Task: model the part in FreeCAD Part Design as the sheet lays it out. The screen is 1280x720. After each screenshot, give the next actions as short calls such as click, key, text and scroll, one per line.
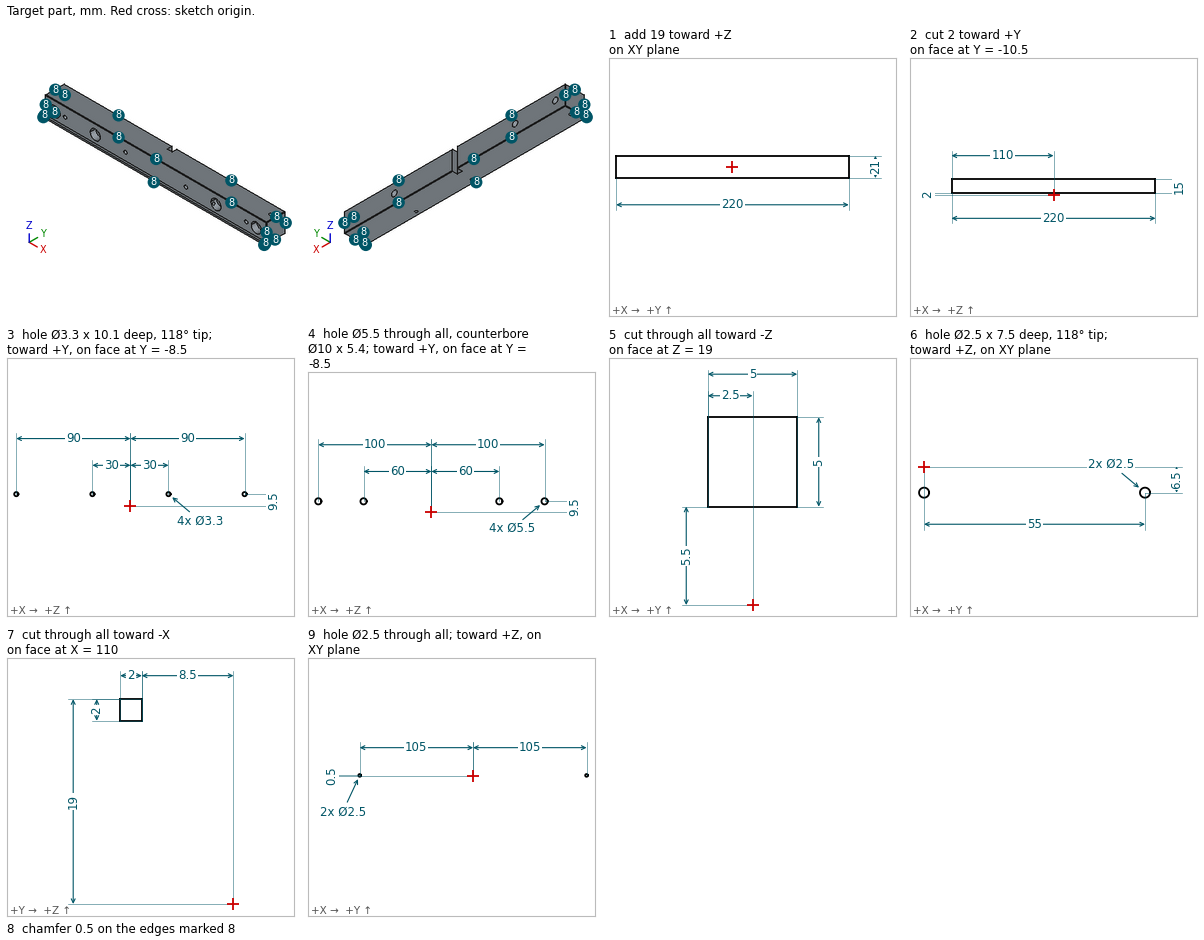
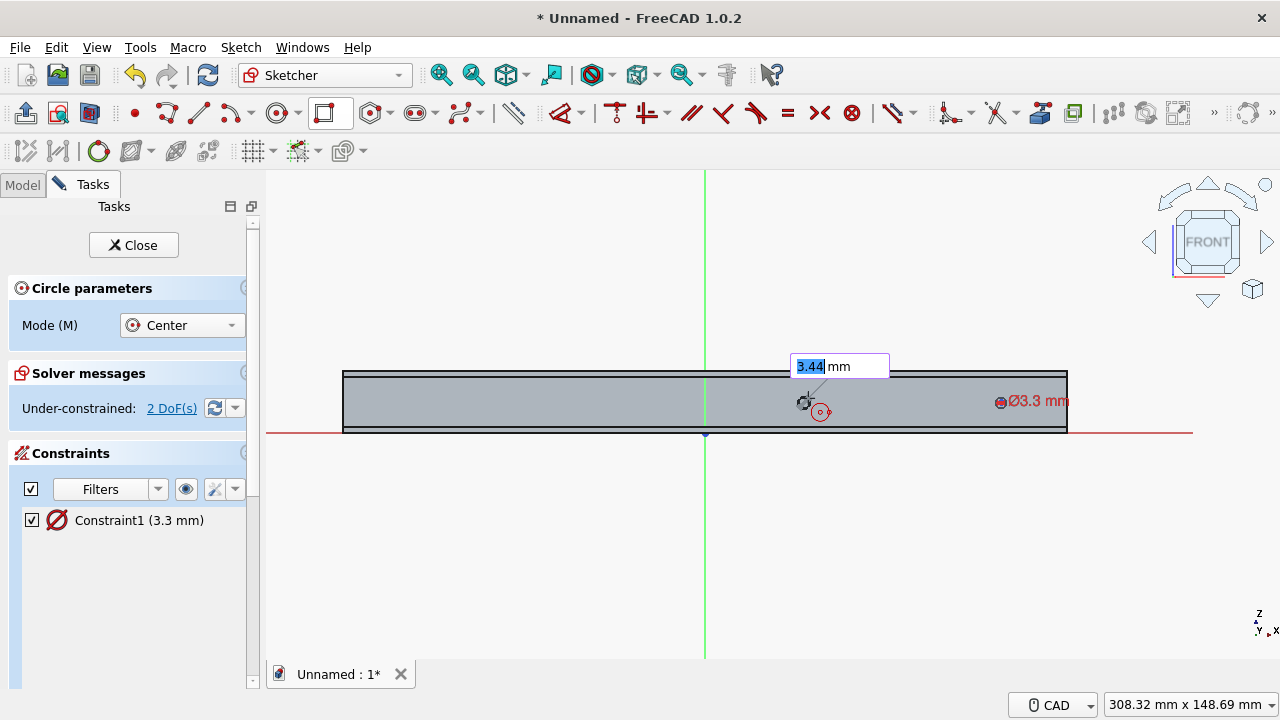
text(3.3)
key(Return)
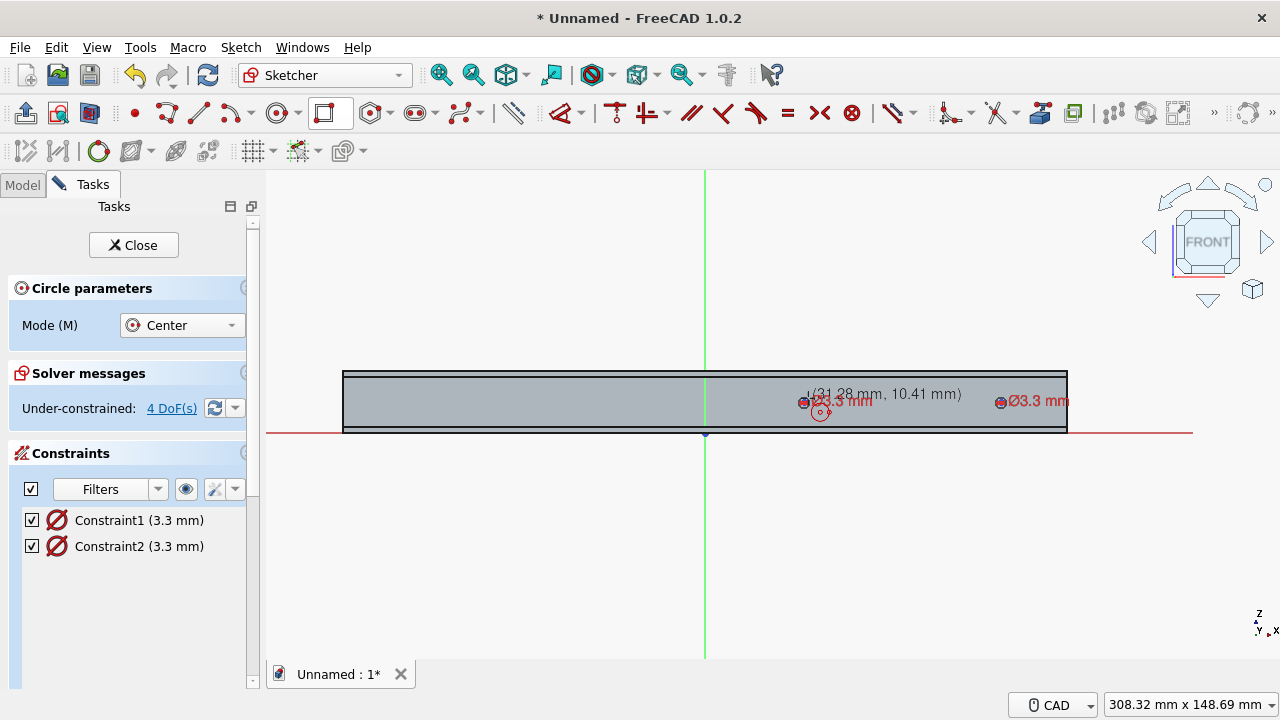
scroll(606, 402, up, 8)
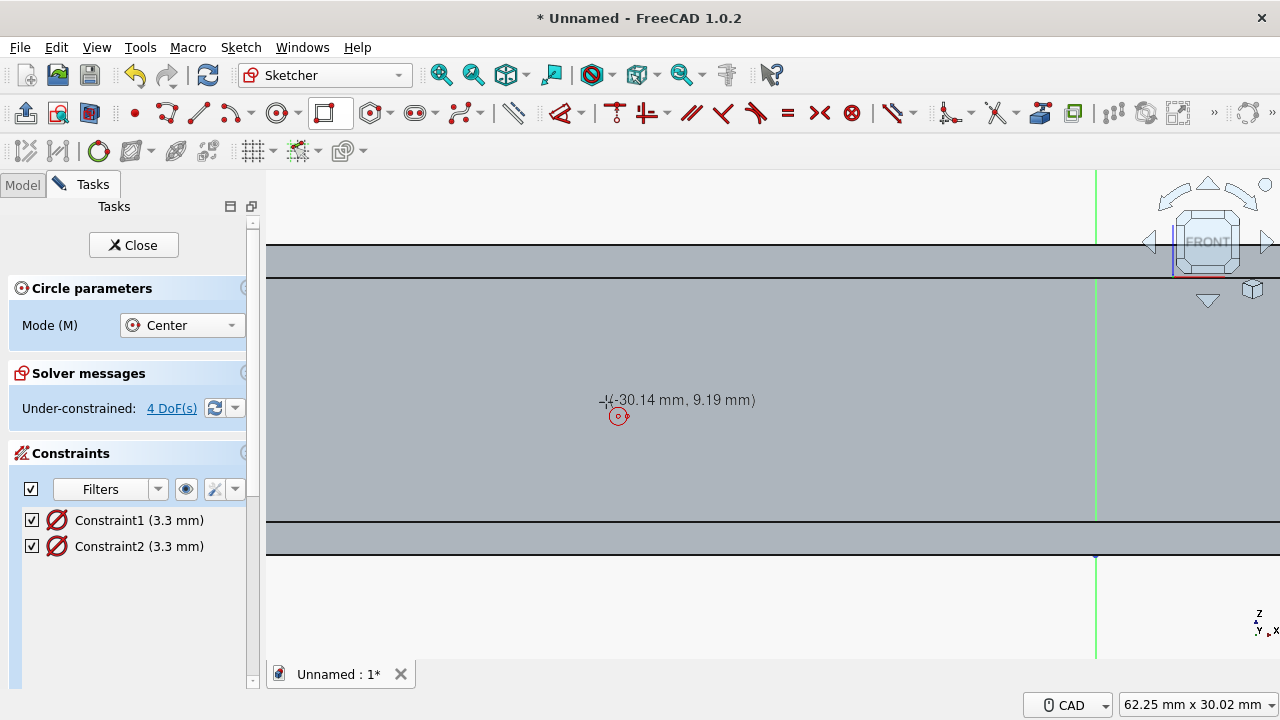
scroll(606, 402, down, 8)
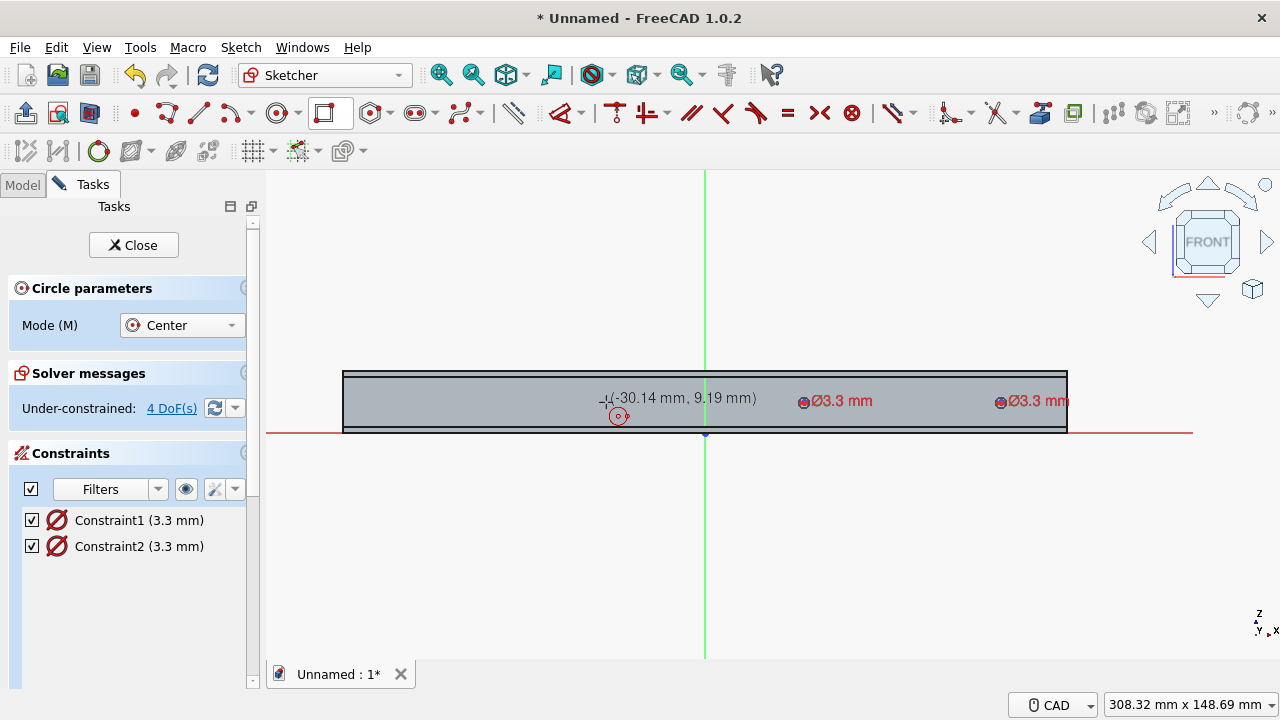
click(606, 402)
move(610, 398)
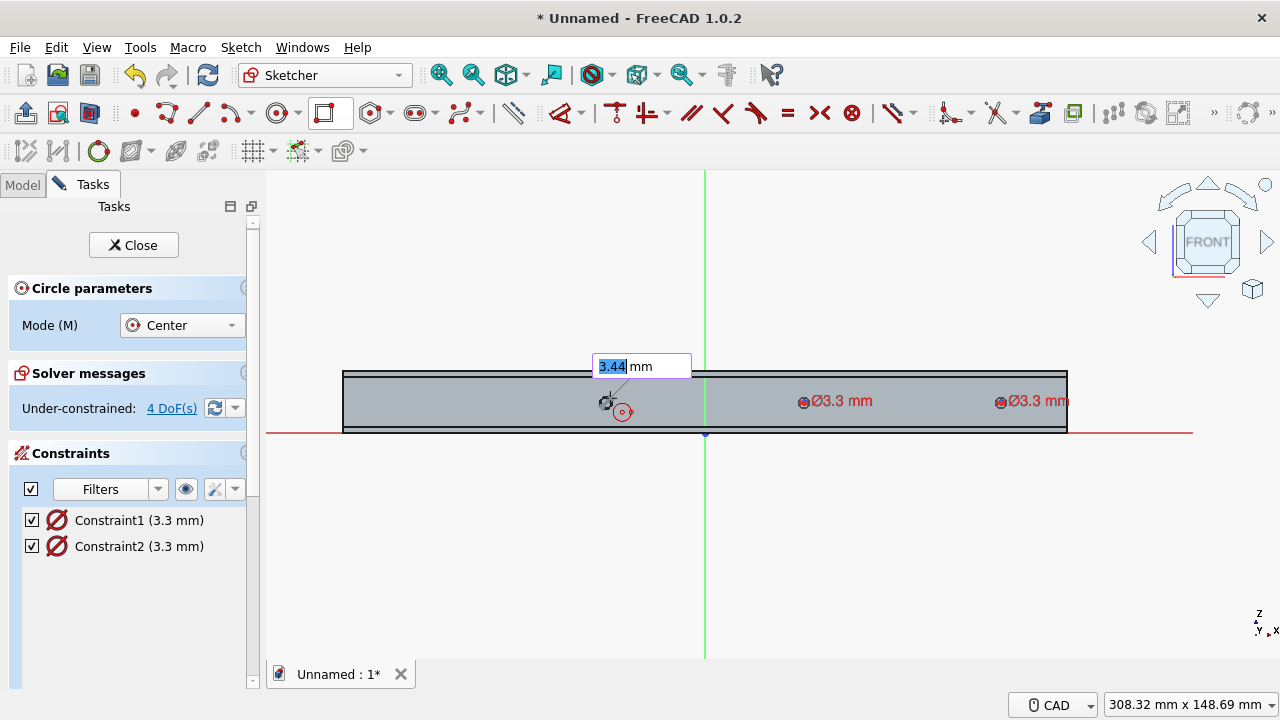
text(3.3)
key(Return)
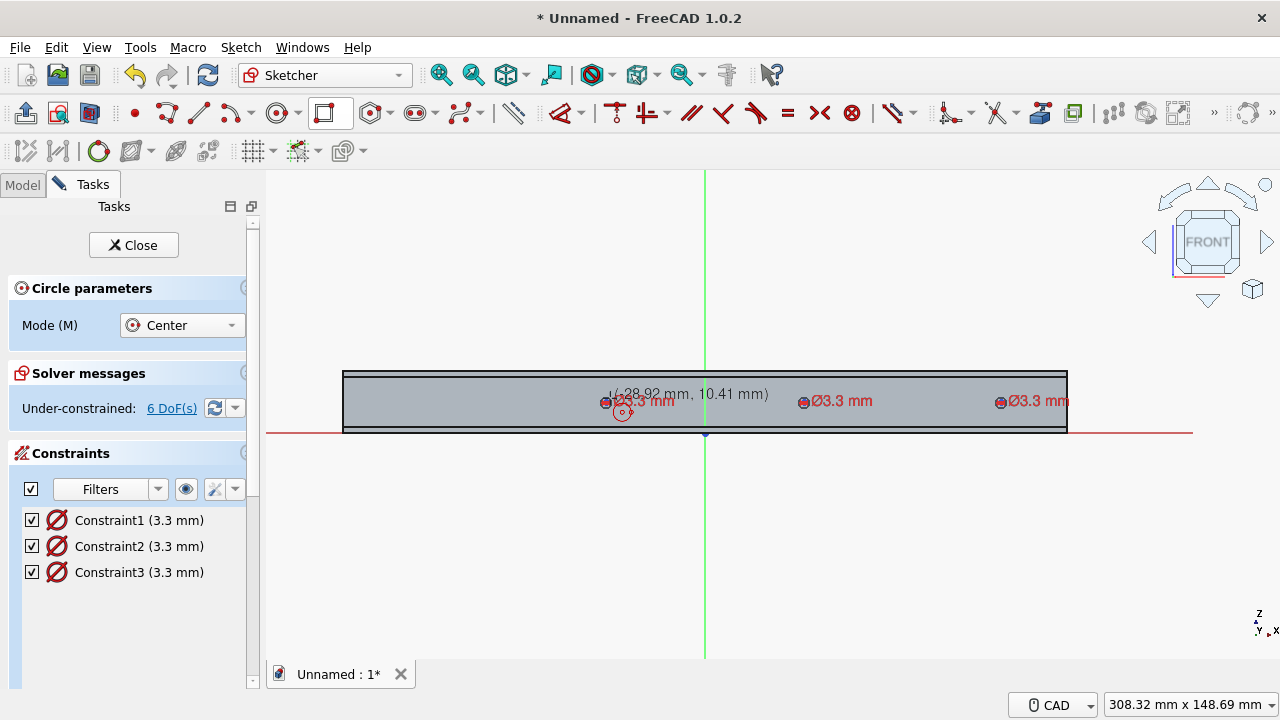
scroll(409, 402, up, 8)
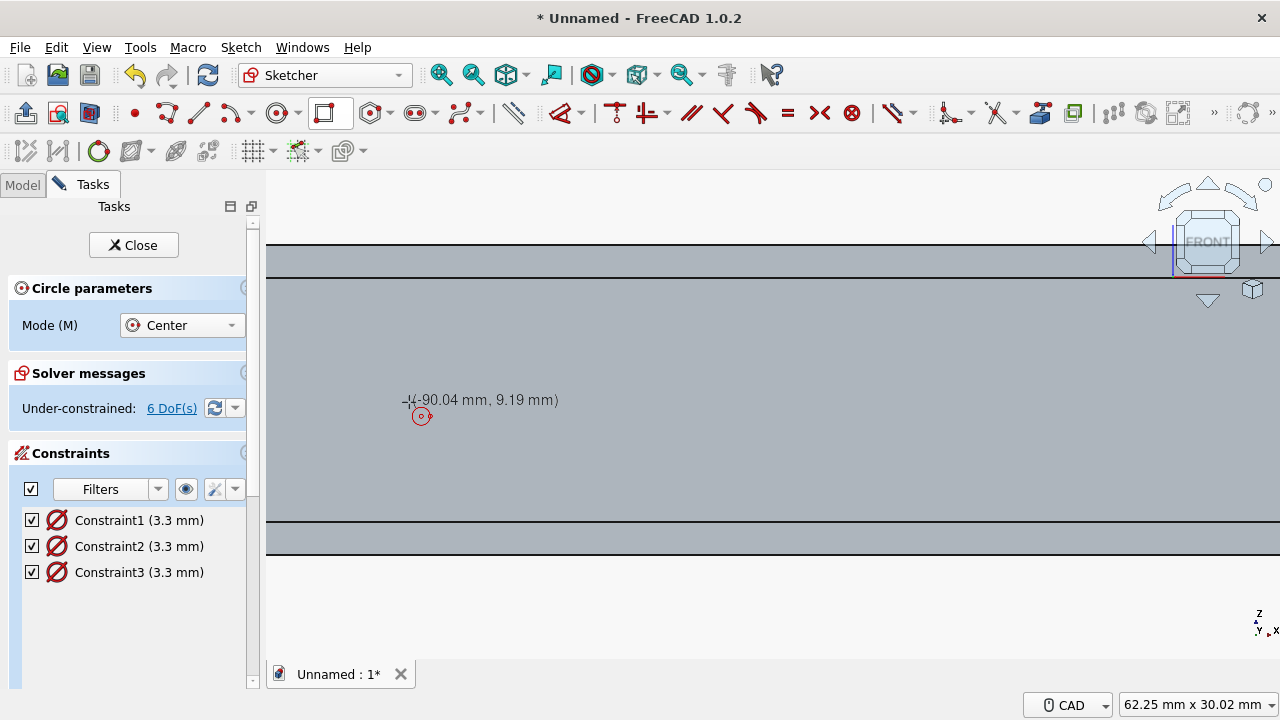
scroll(408, 402, down, 8)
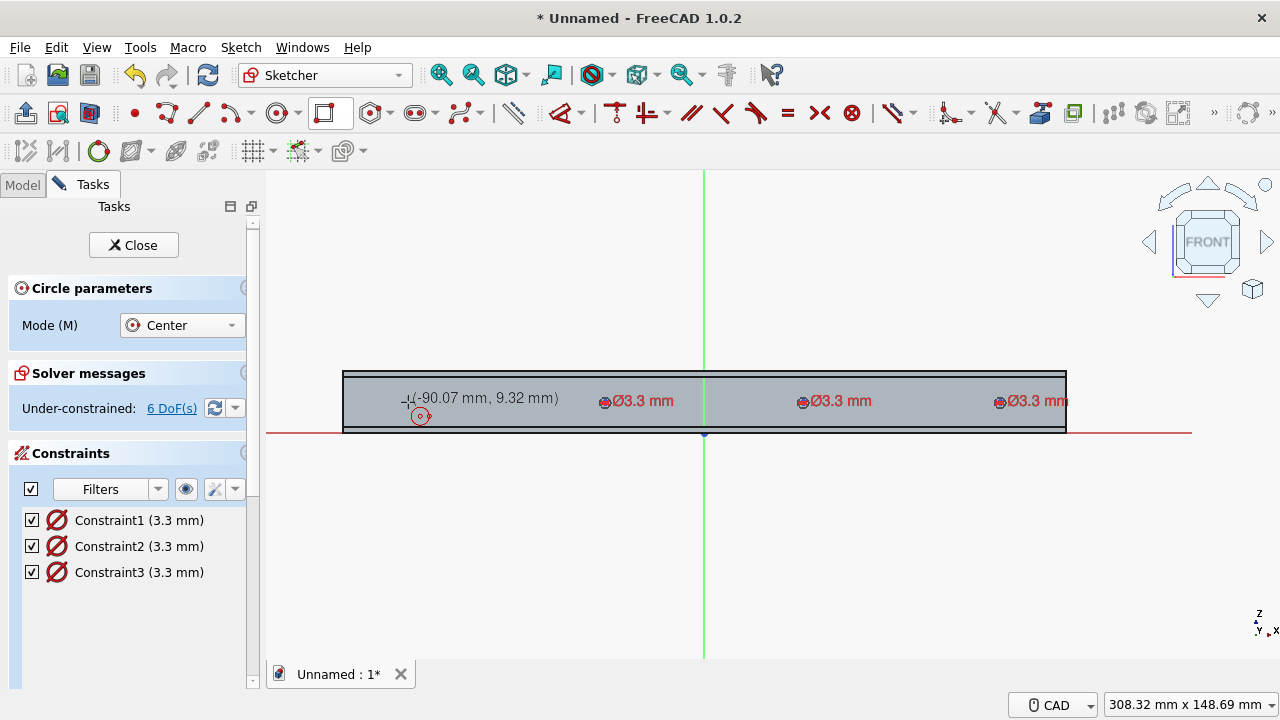
click(408, 402)
move(412, 398)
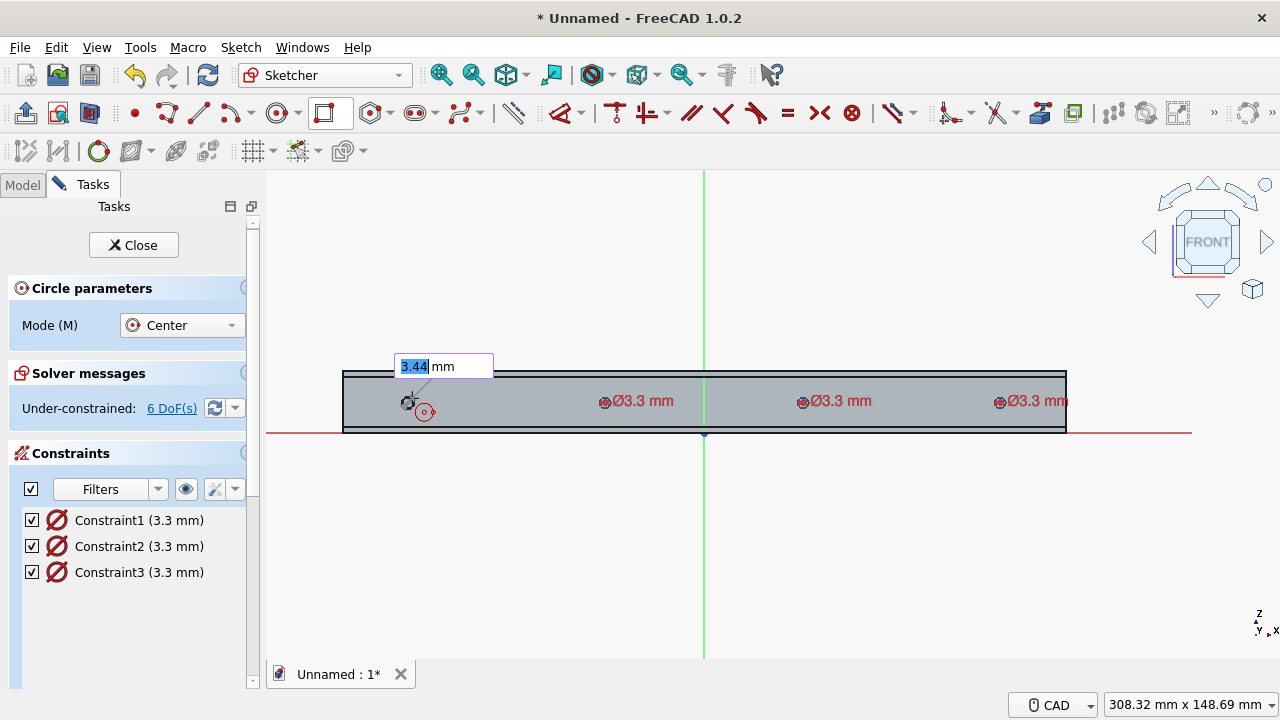
text(3.3)
key(Return)
key(Escape)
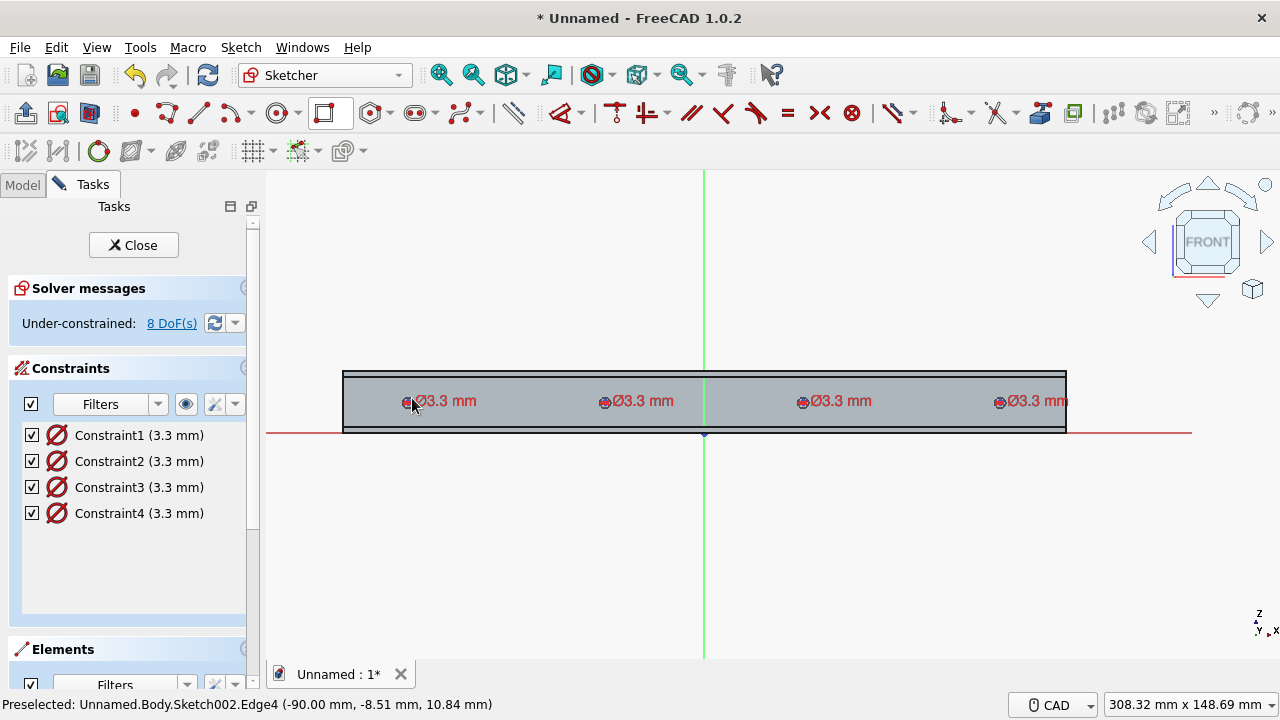
click(1000, 403)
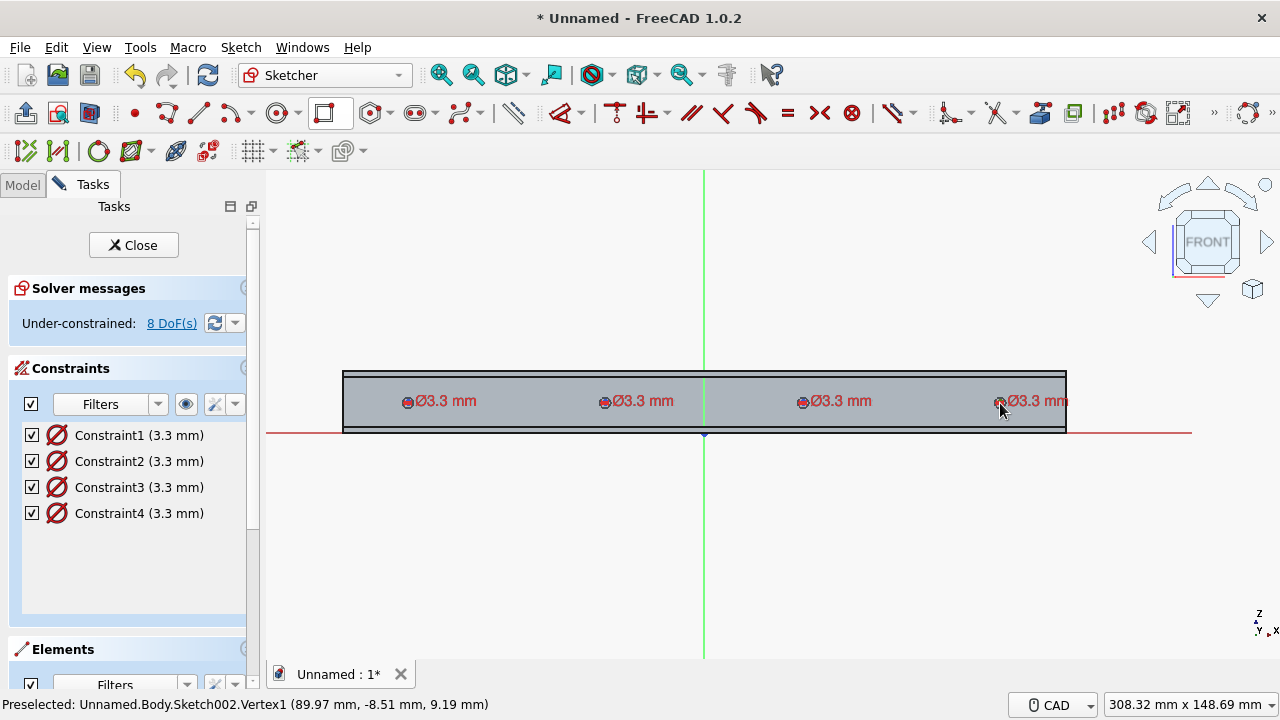
click(803, 403)